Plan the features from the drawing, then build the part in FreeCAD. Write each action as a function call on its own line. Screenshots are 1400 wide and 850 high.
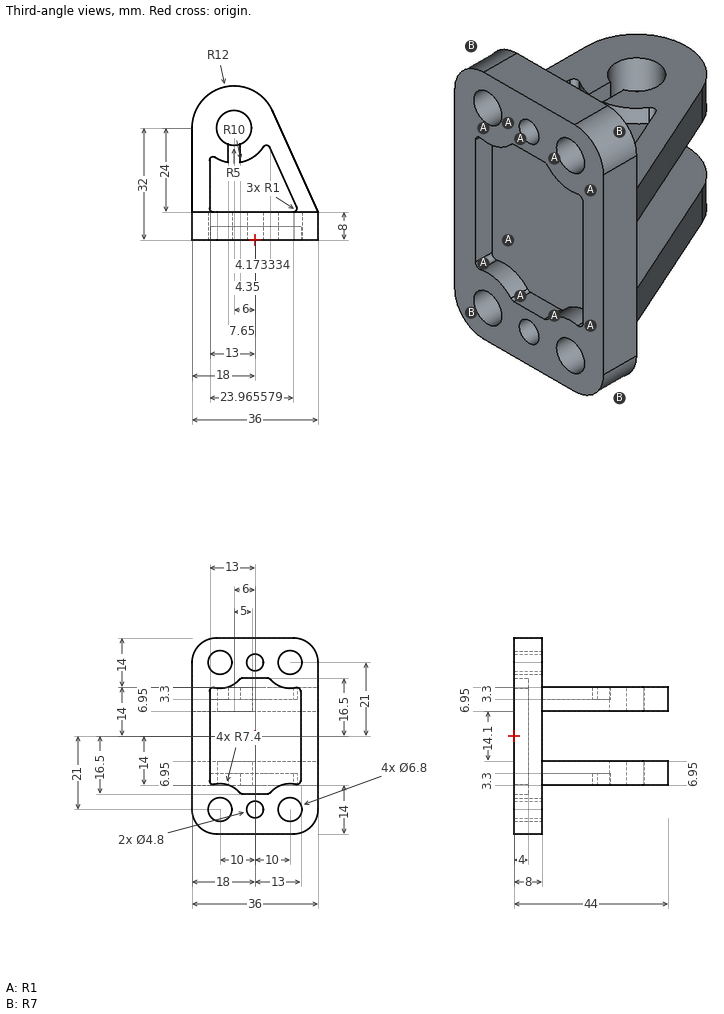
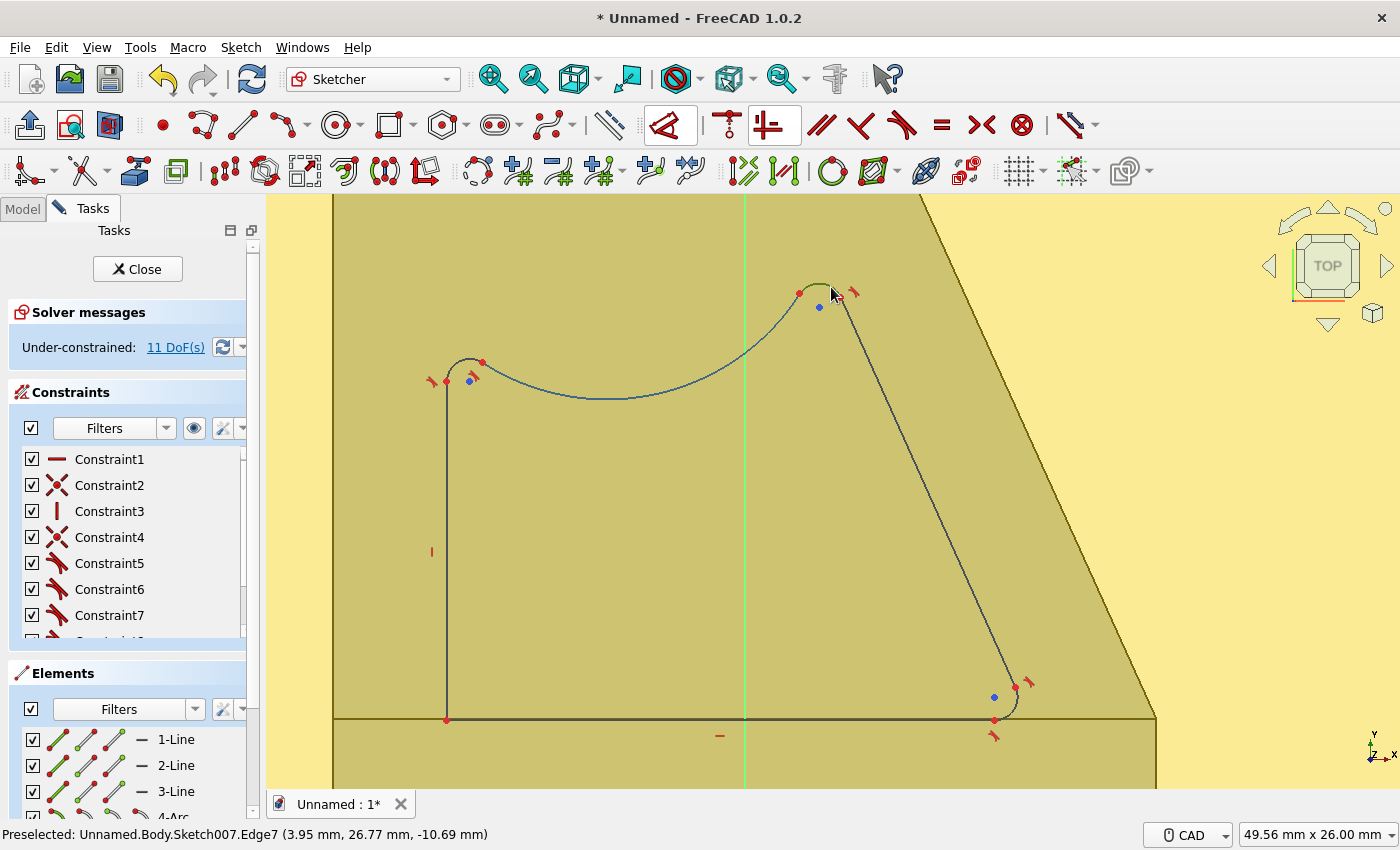
click(902, 126)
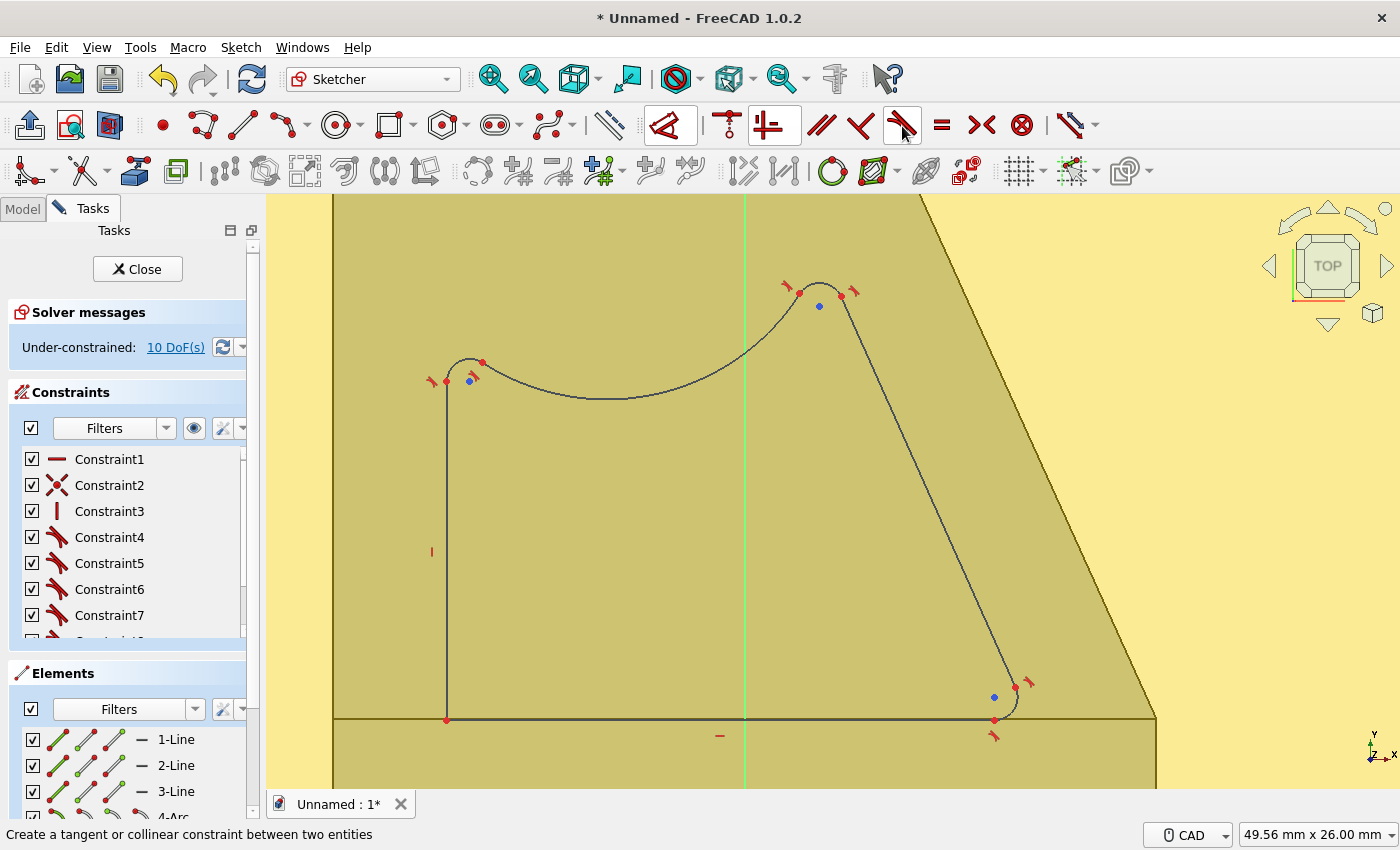
click(1007, 716)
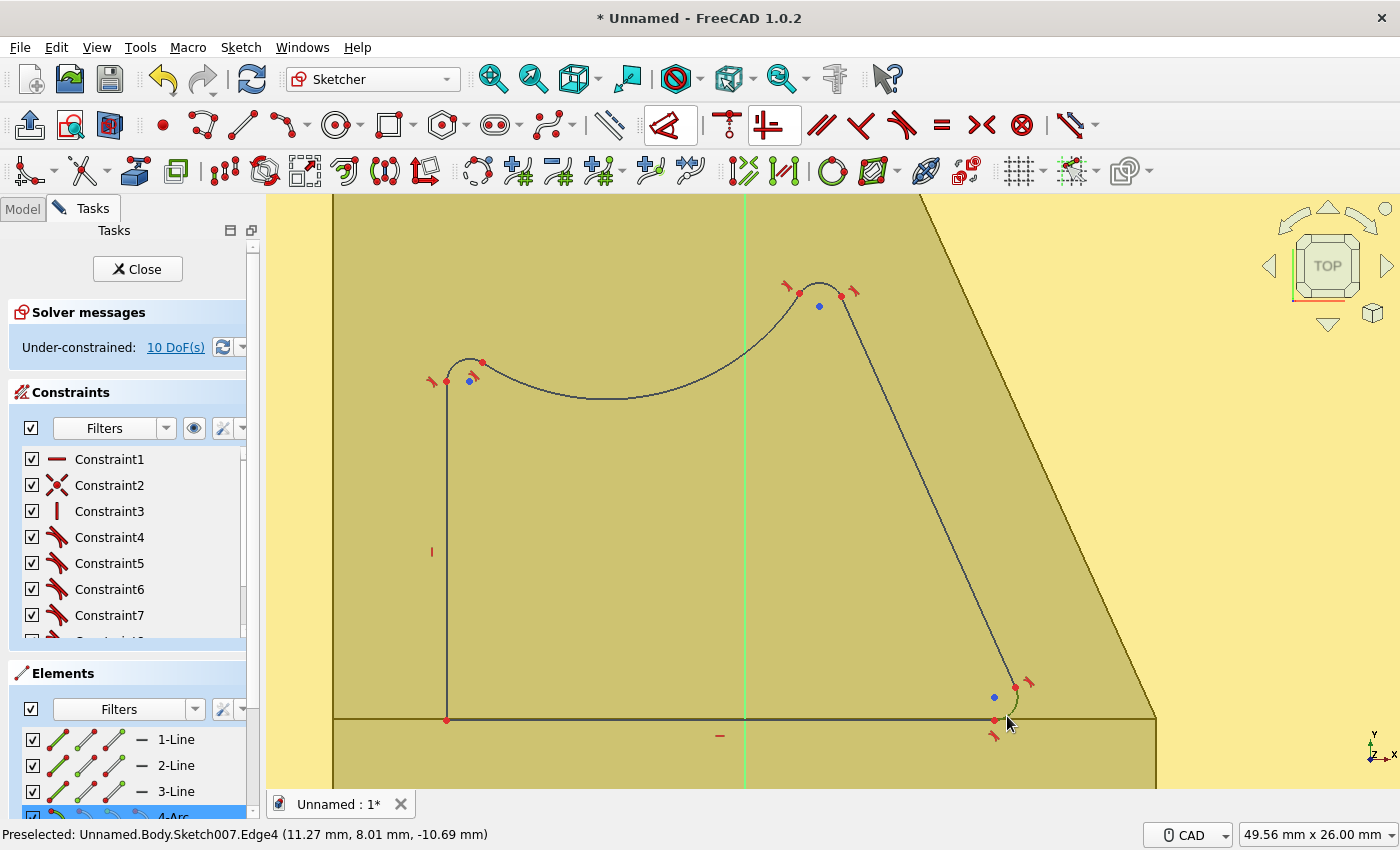
click(468, 359)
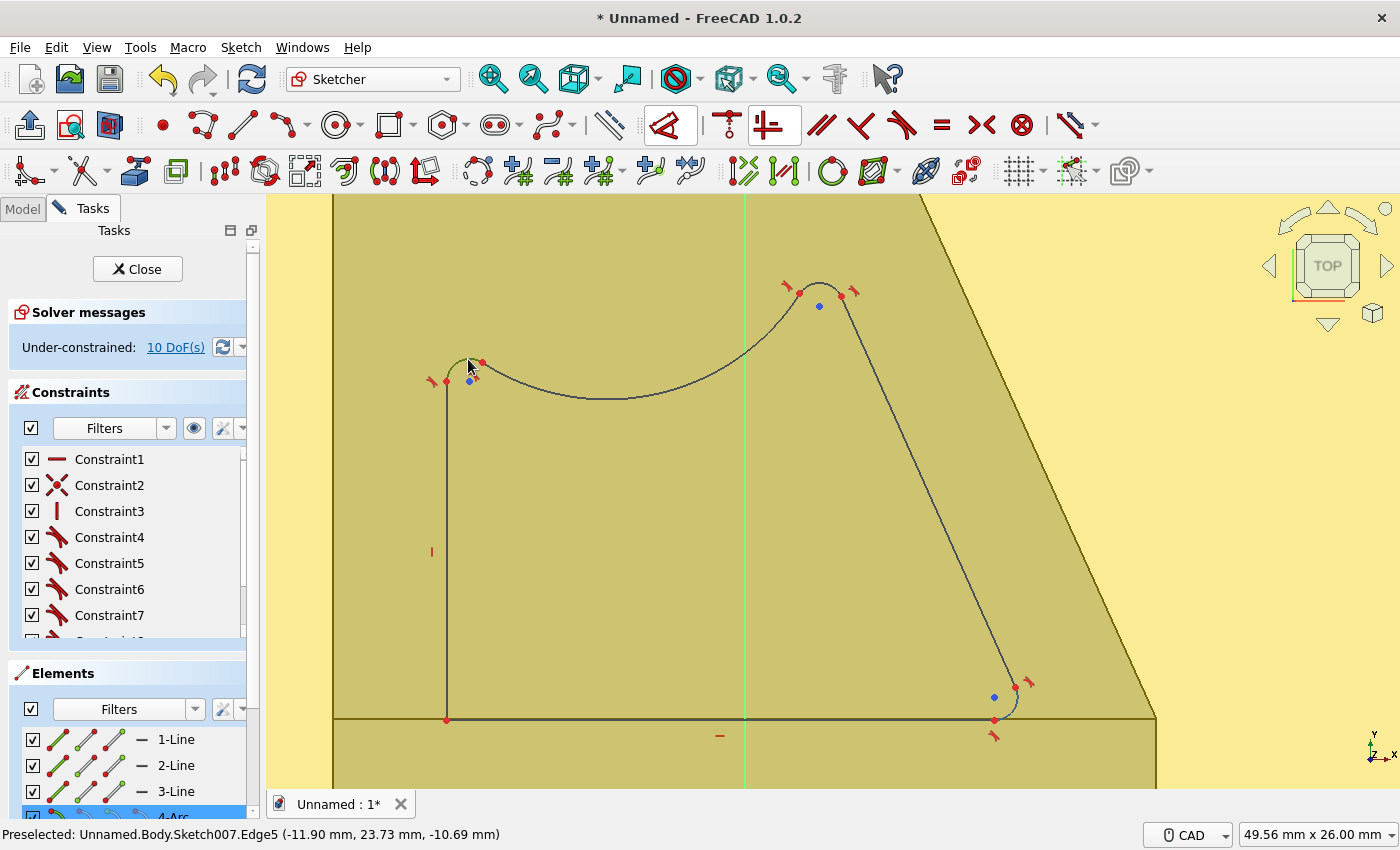
click(831, 286)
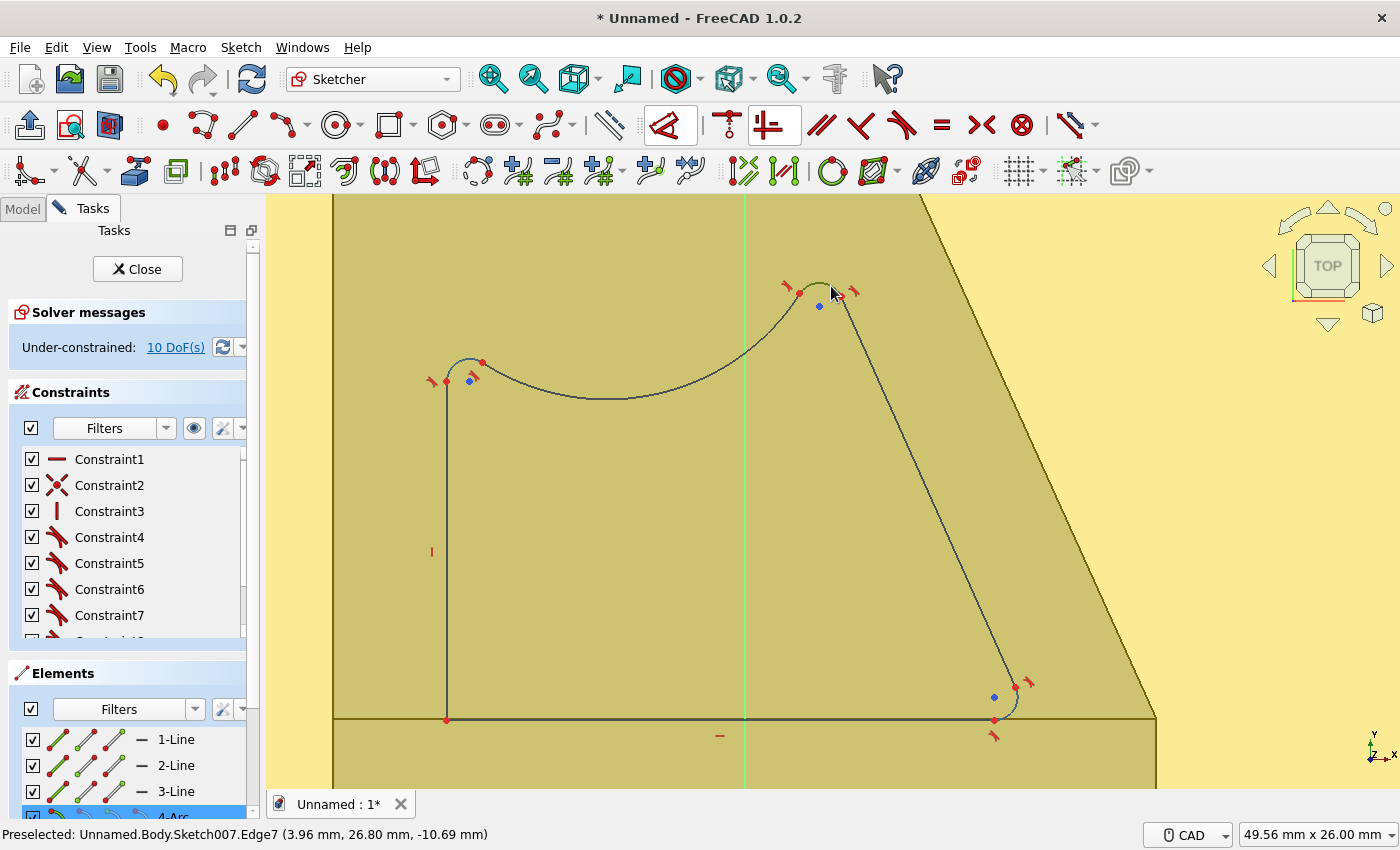
key(e)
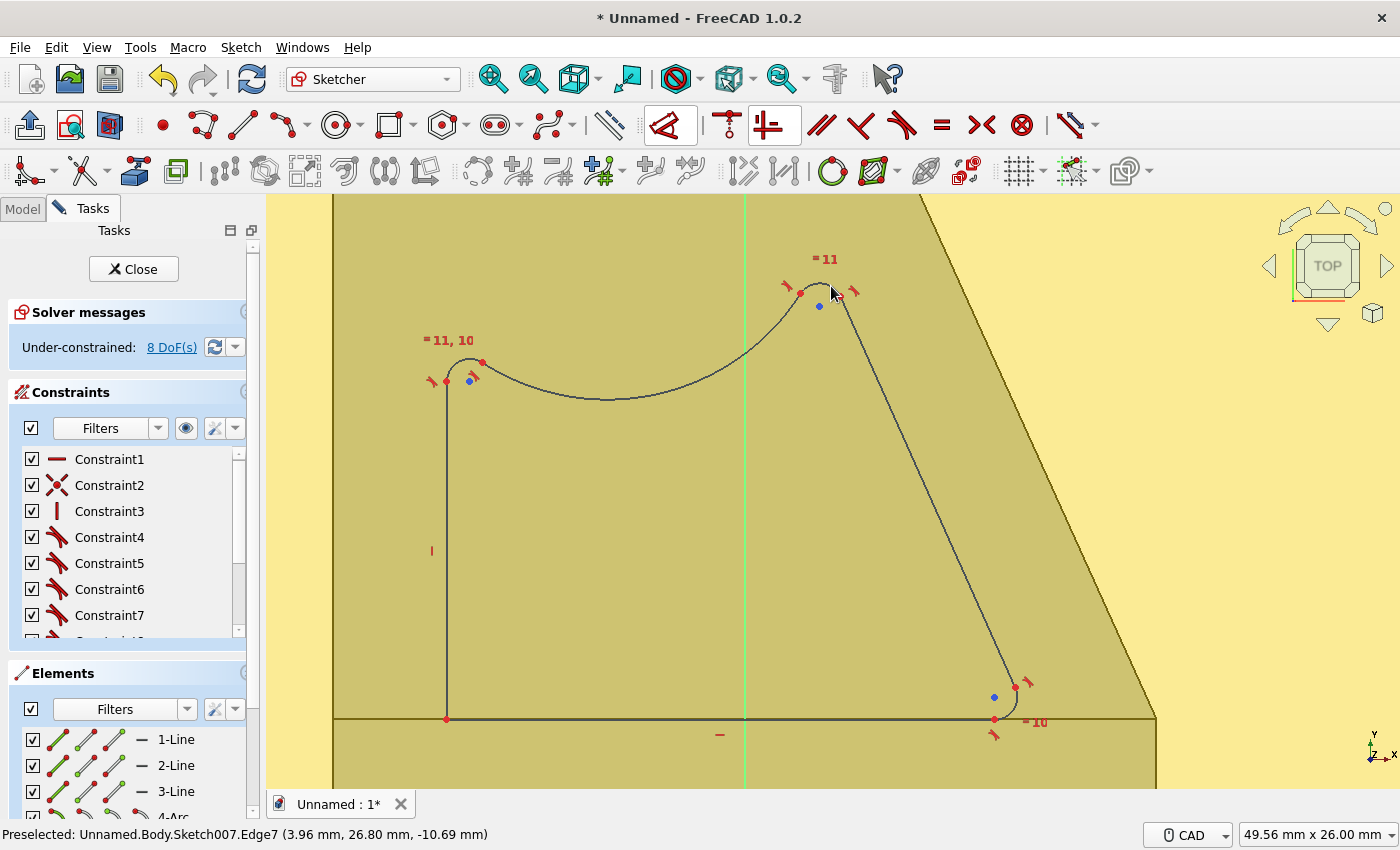
scroll(1007, 716, up, 3)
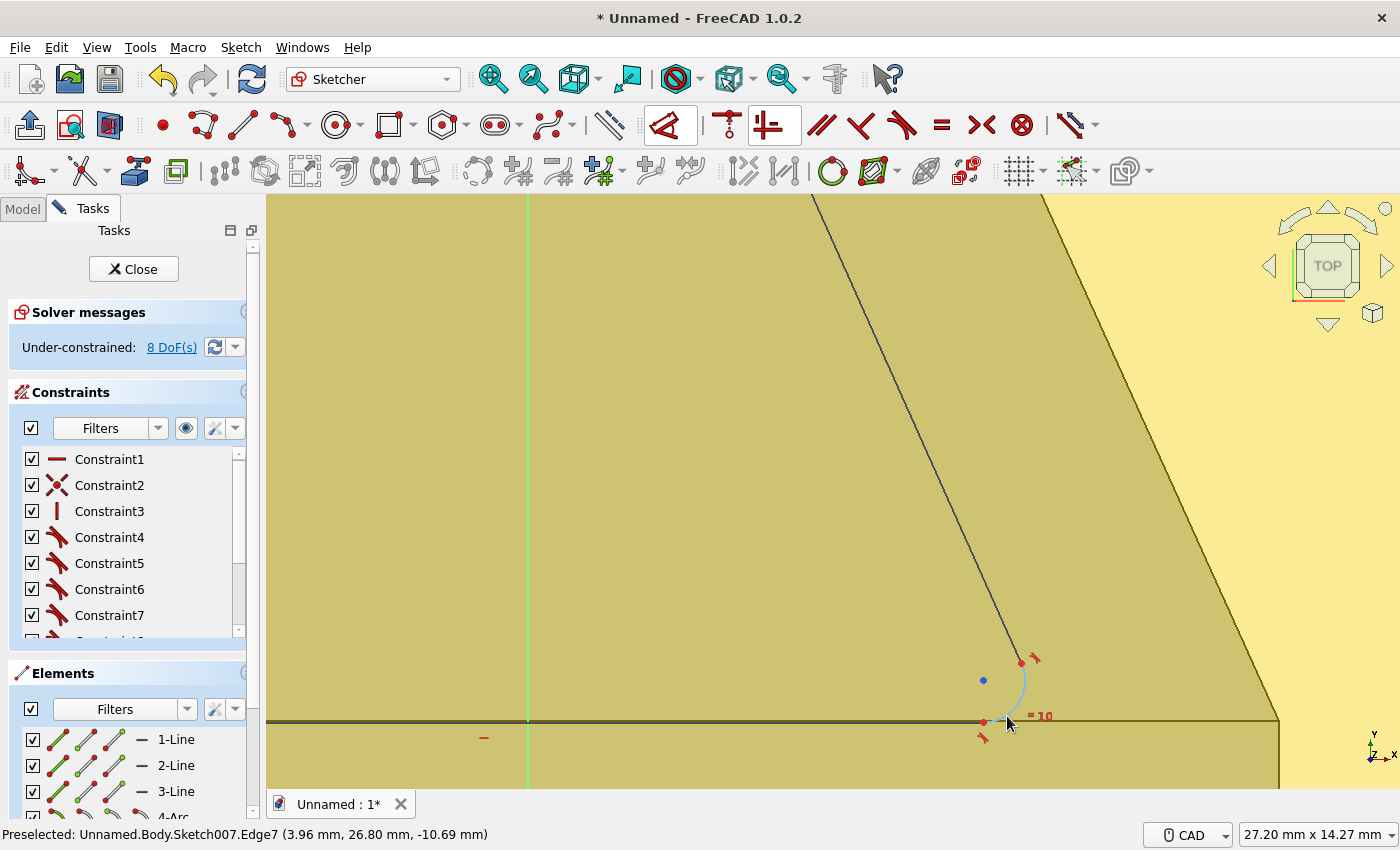
click(1007, 715)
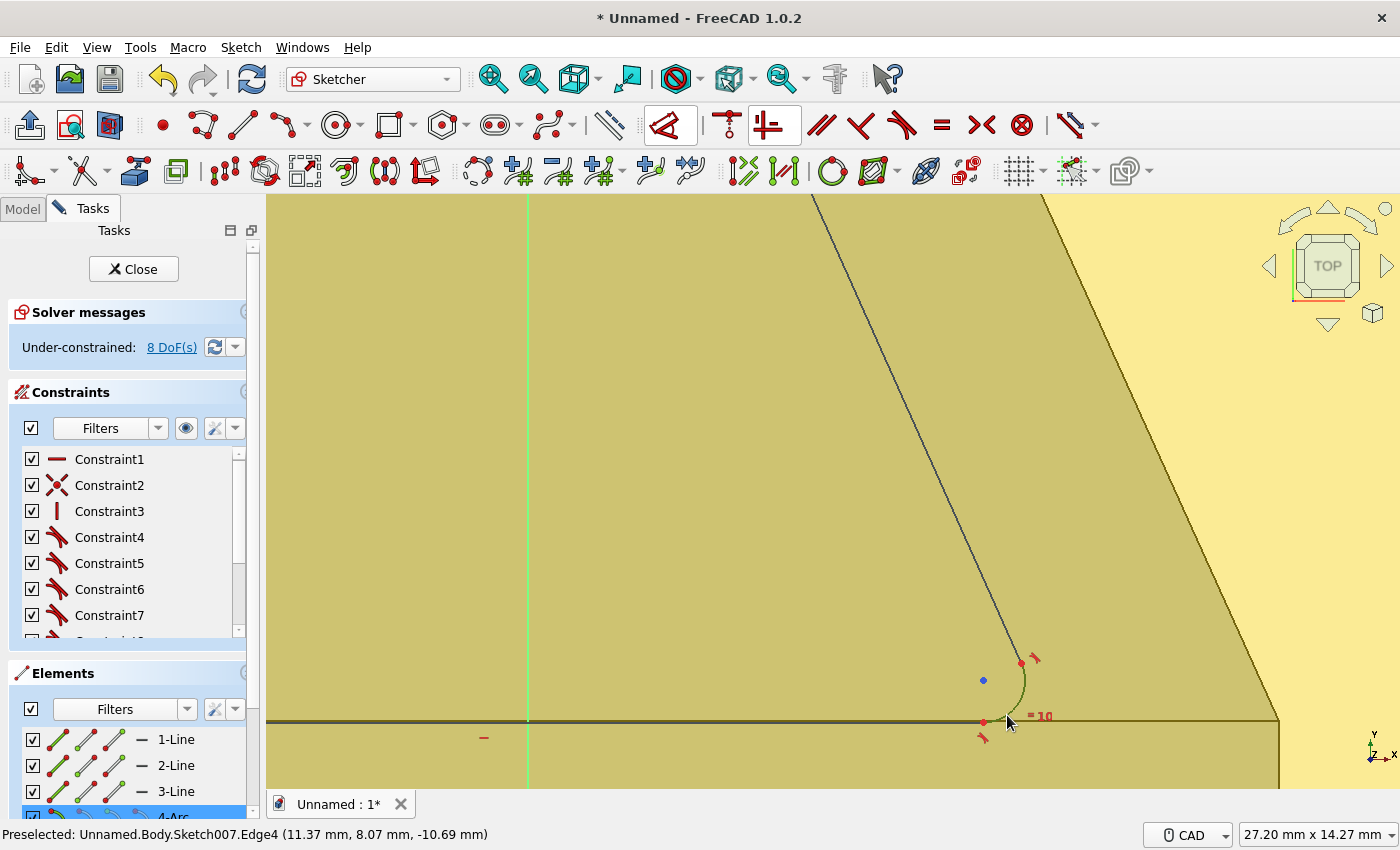
click(692, 126)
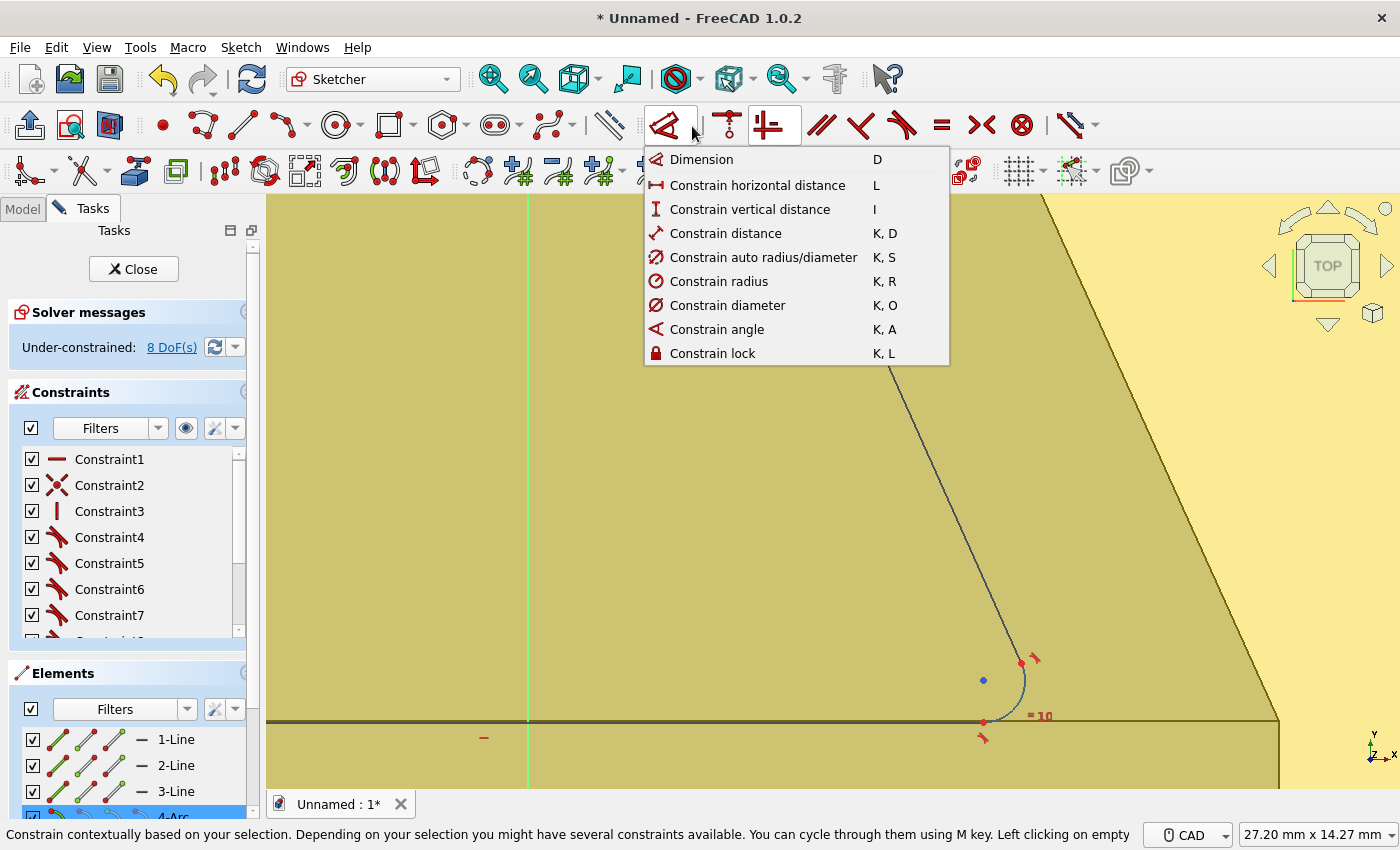
click(797, 281)